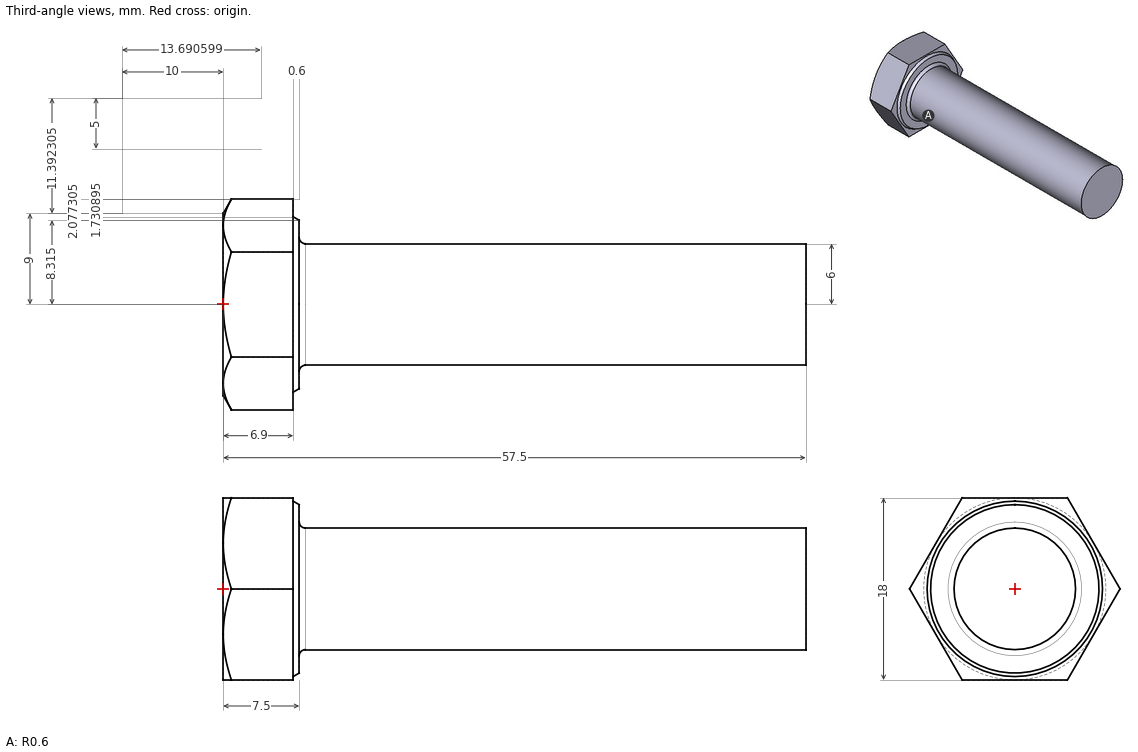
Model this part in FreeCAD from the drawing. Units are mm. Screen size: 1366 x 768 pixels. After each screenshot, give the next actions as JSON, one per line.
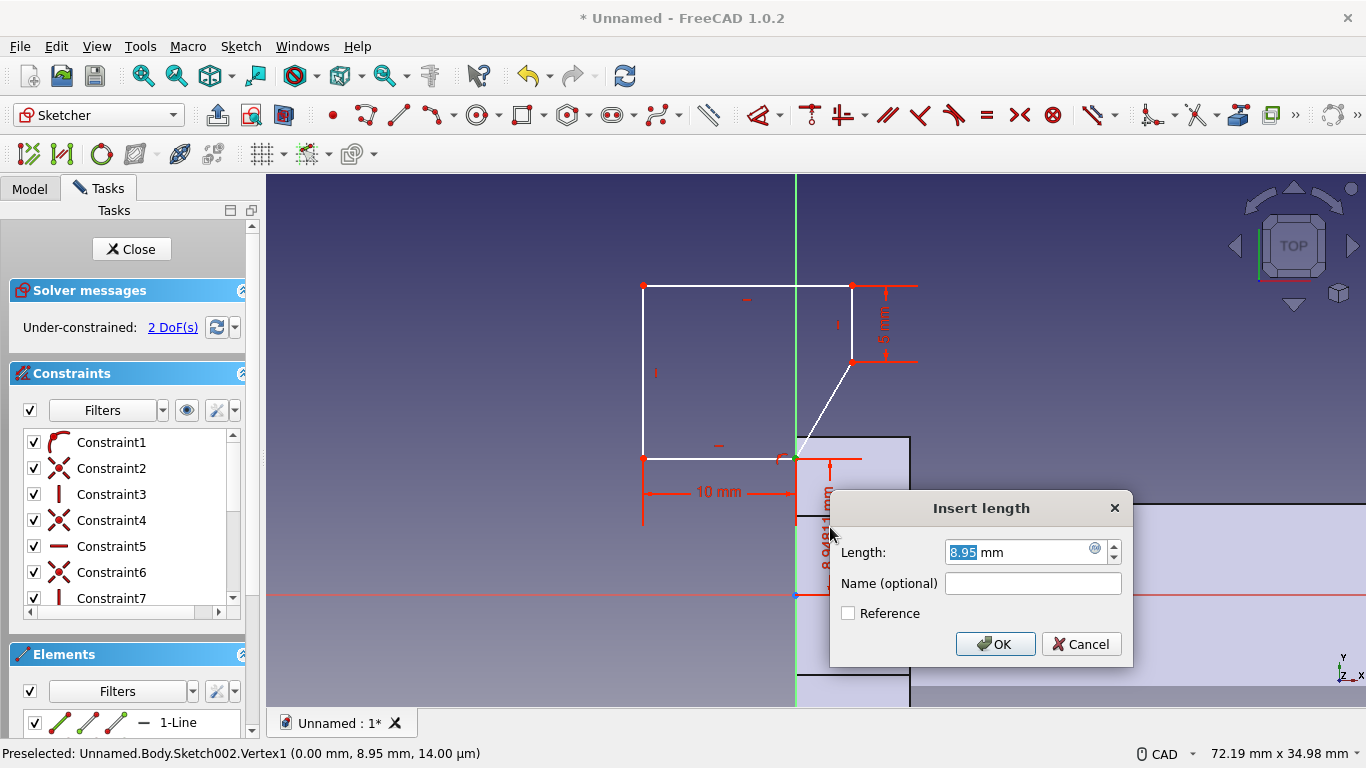
{"action": "type", "text": "9"}
{"action": "key", "text": "Return"}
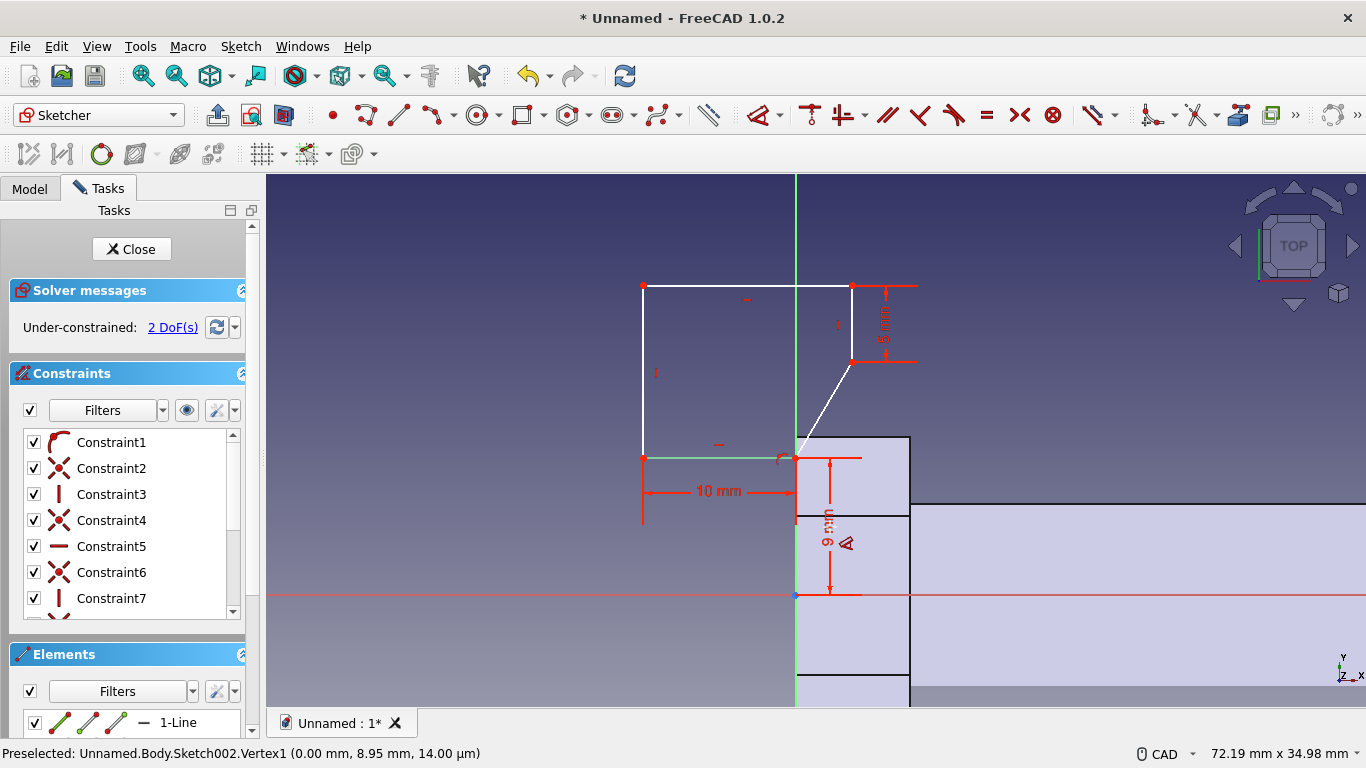
{"action": "left_click", "coordinate": [706, 286]}
{"action": "left_click", "coordinate": [748, 252]}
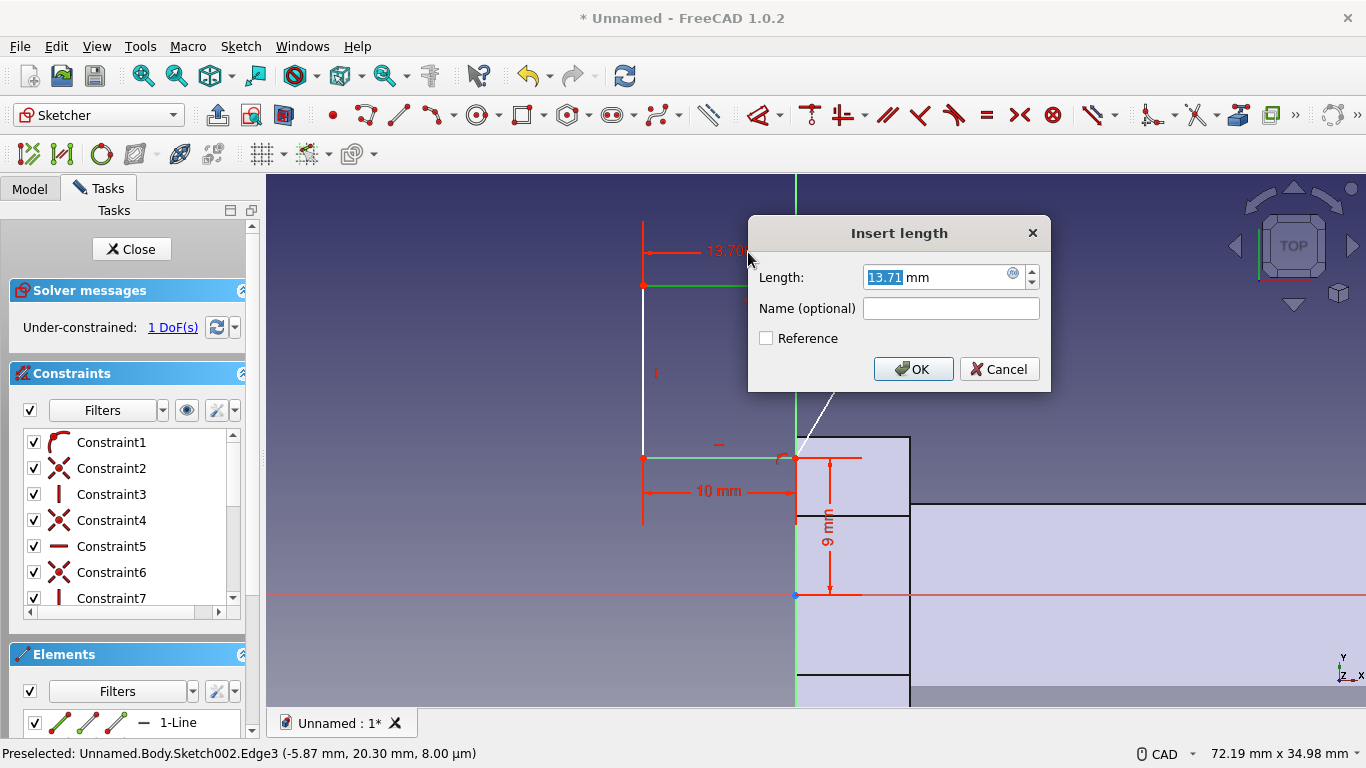
{"action": "type", "text": "13.690599"}
{"action": "key", "text": "Return"}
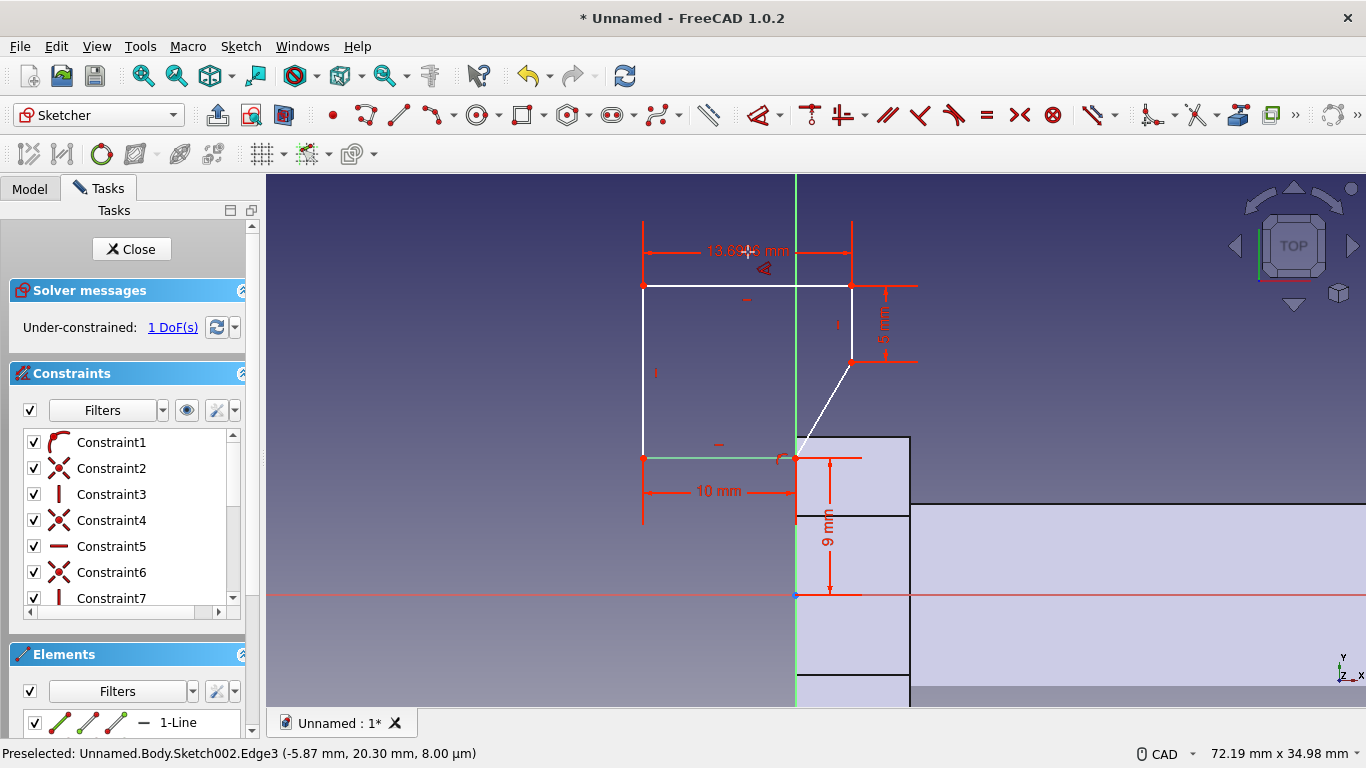
{"action": "left_click", "coordinate": [643, 338]}
{"action": "left_click", "coordinate": [609, 372]}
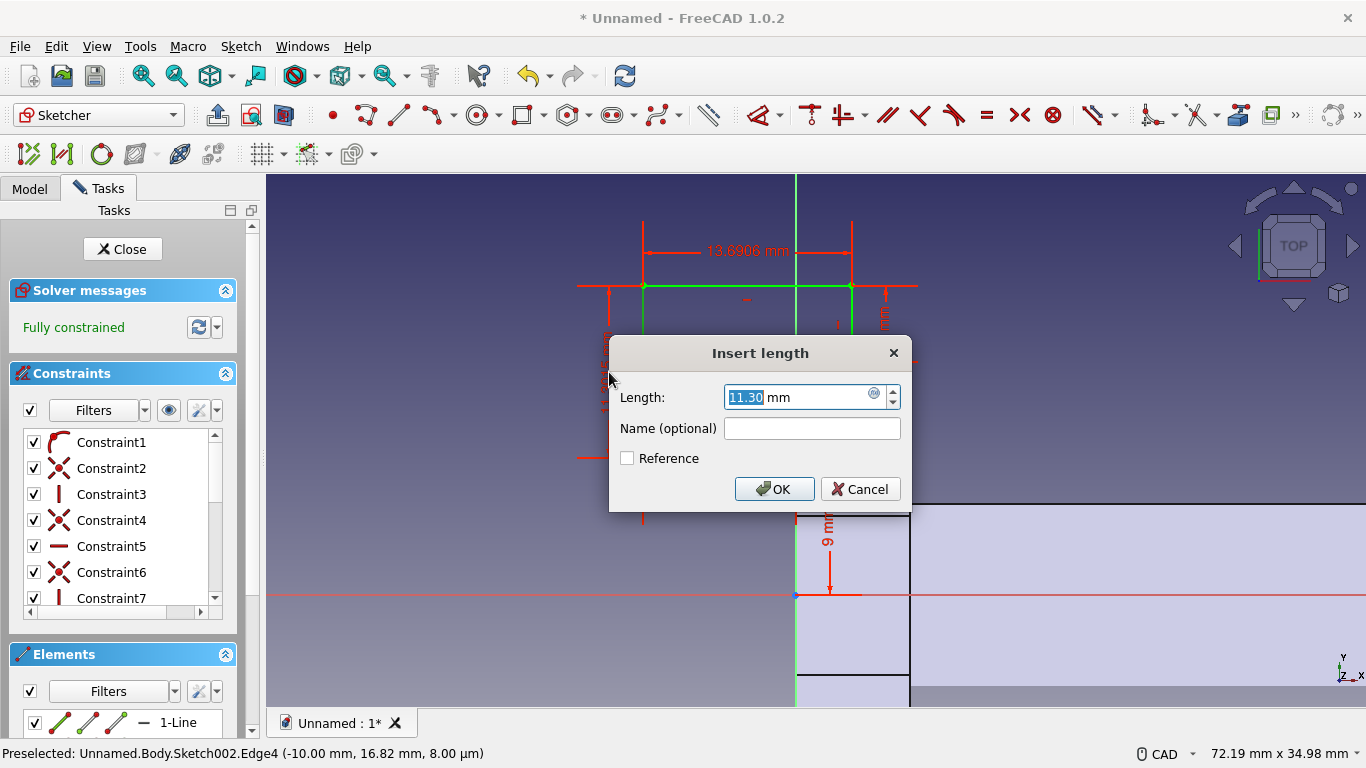
{"action": "type", "text": "11.392305"}
{"action": "key", "text": "Return"}
{"action": "key", "text": "Escape"}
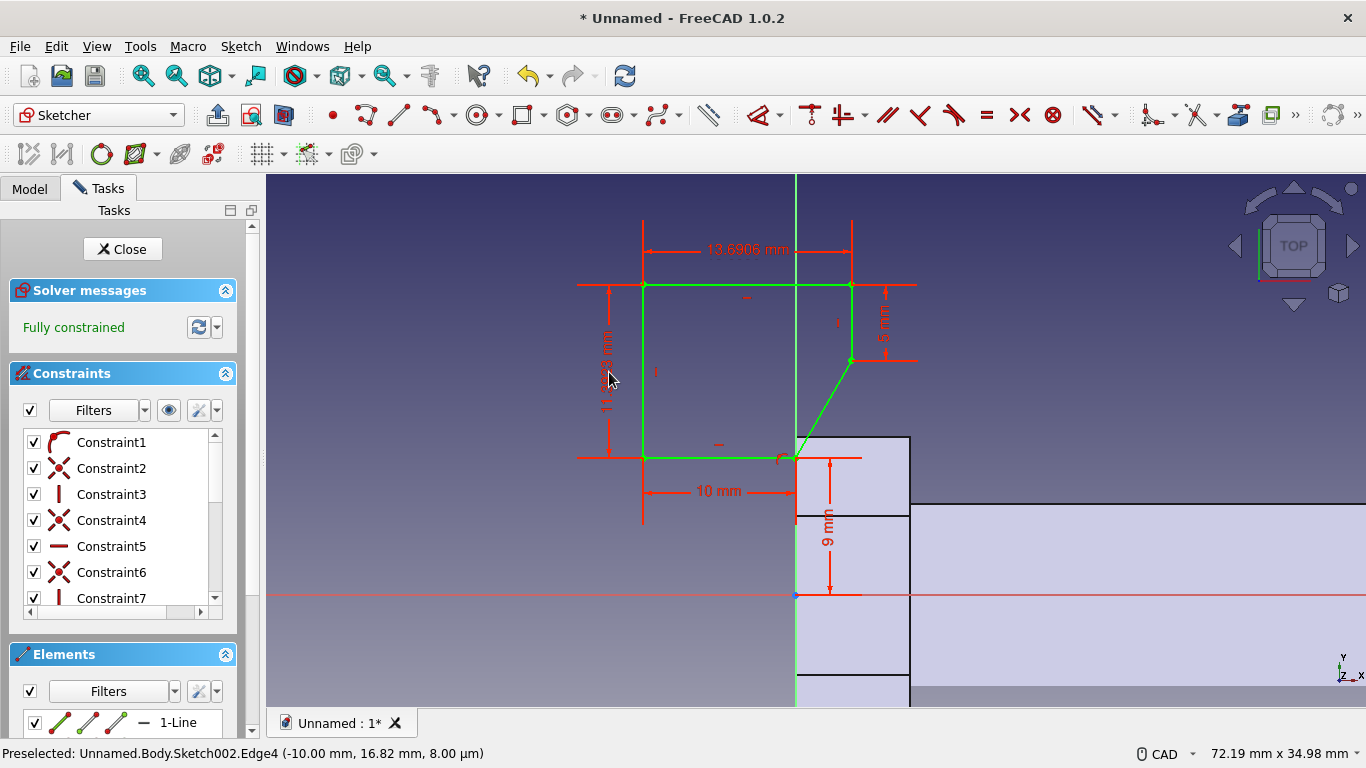
{"action": "left_click", "coordinate": [123, 249]}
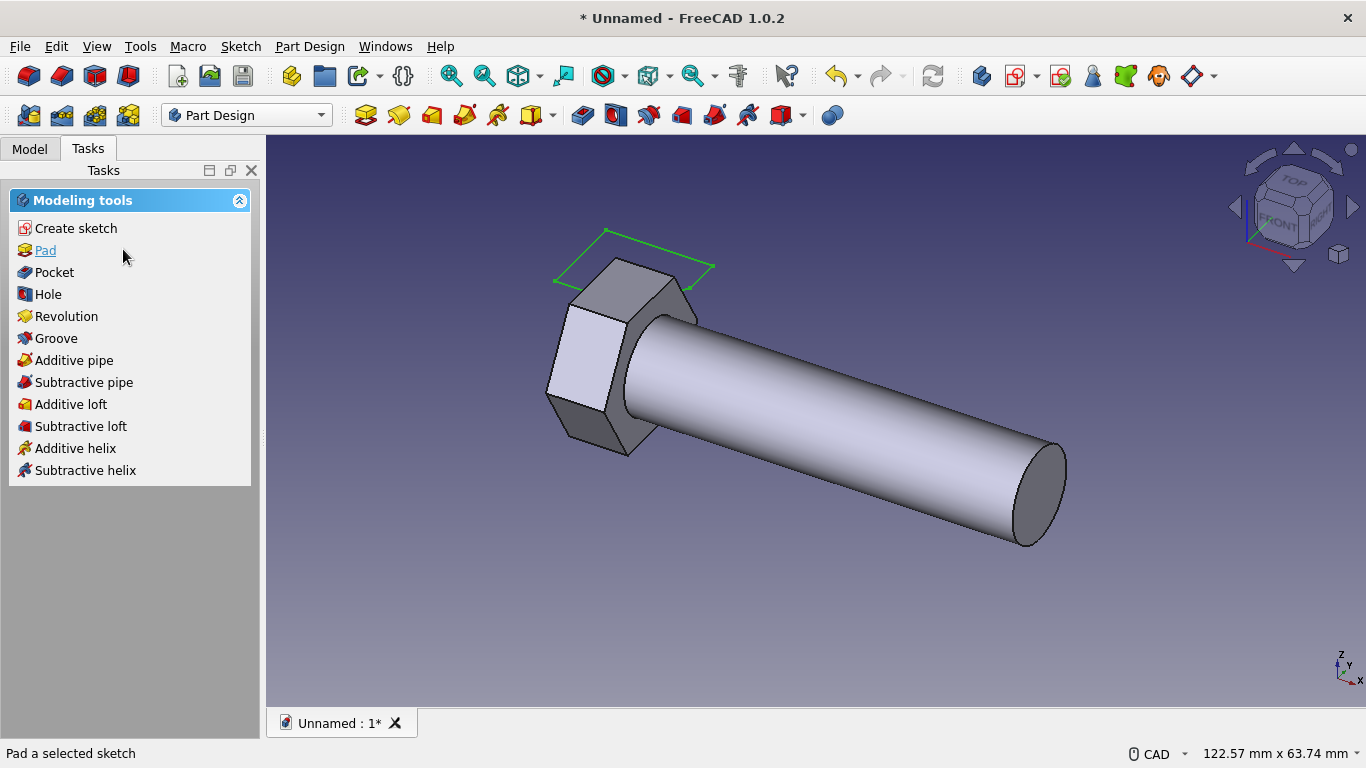
{"action": "left_click", "coordinate": [649, 116]}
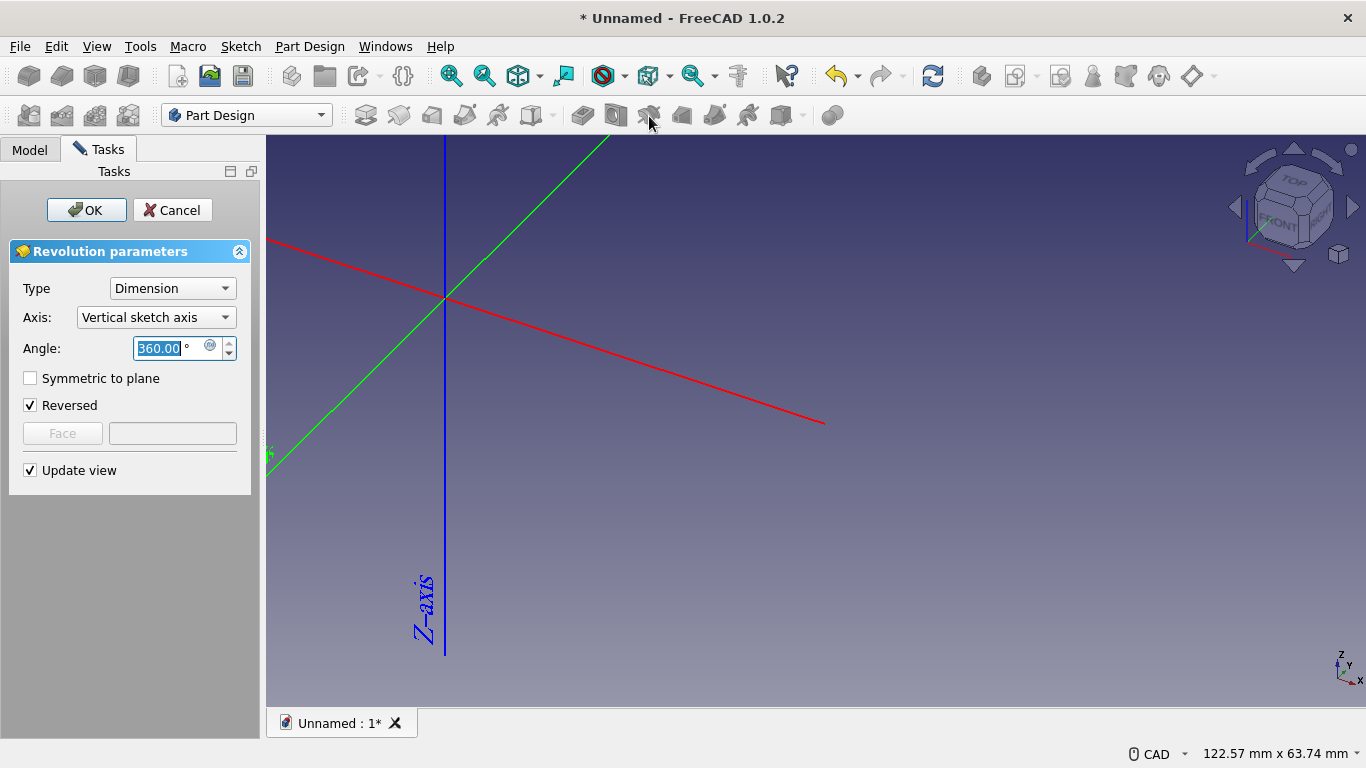
{"action": "left_click", "coordinate": [157, 318]}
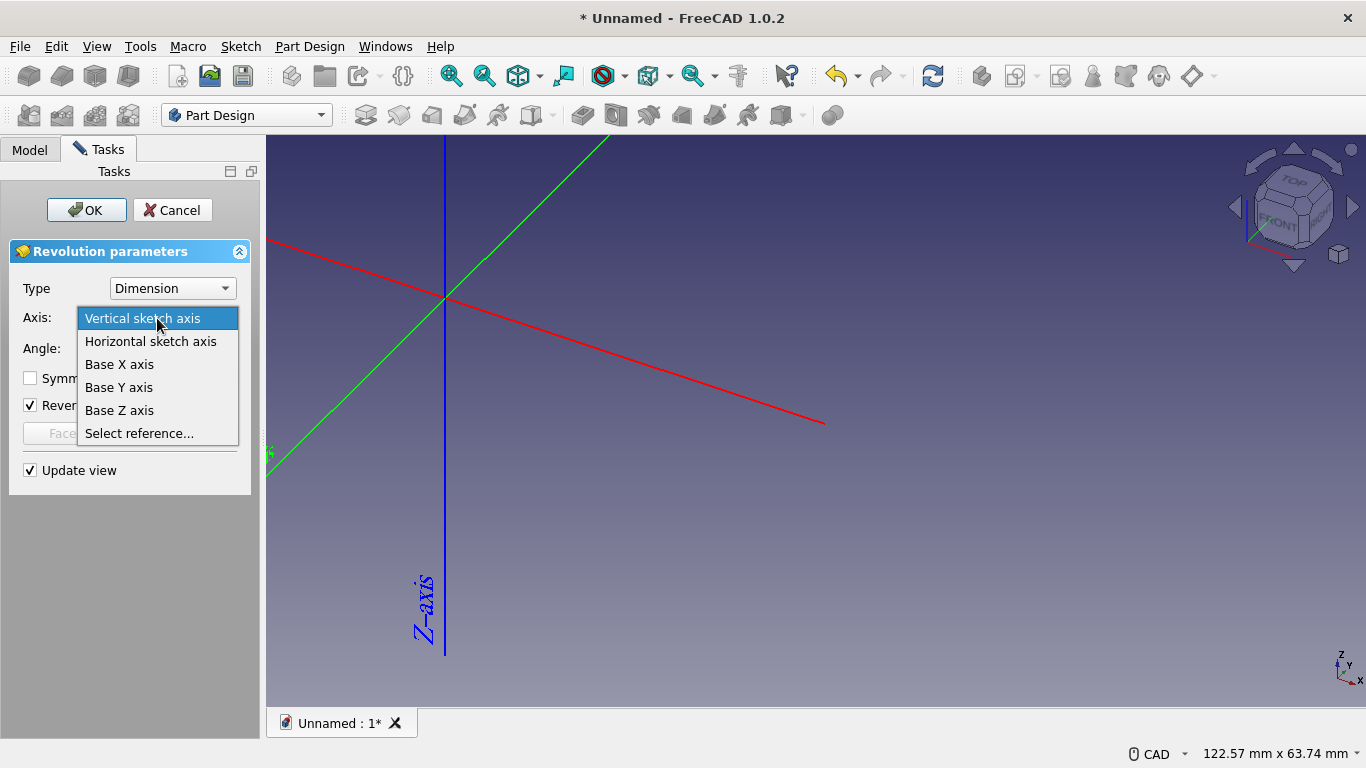
{"action": "left_click", "coordinate": [156, 342]}